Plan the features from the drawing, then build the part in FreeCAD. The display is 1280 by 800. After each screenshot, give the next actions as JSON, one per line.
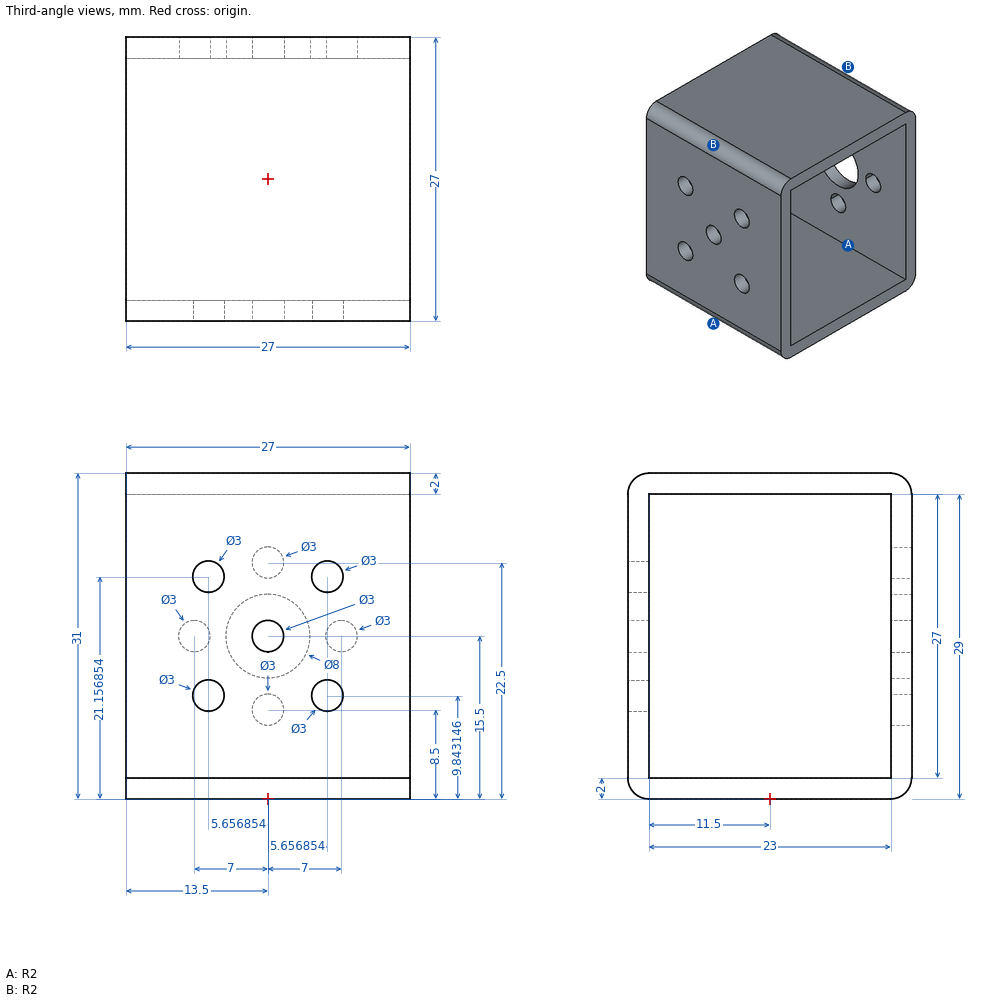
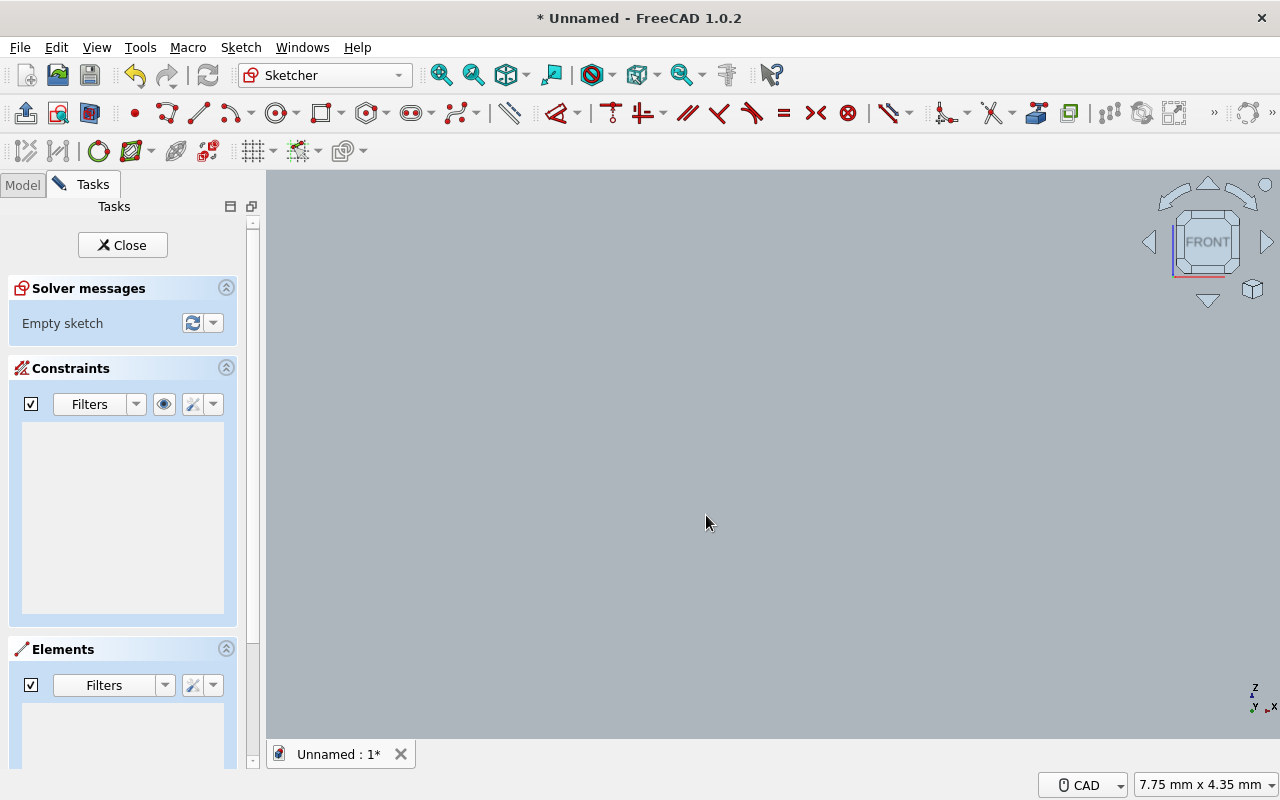
{"action": "left_click", "coordinate": [276, 114]}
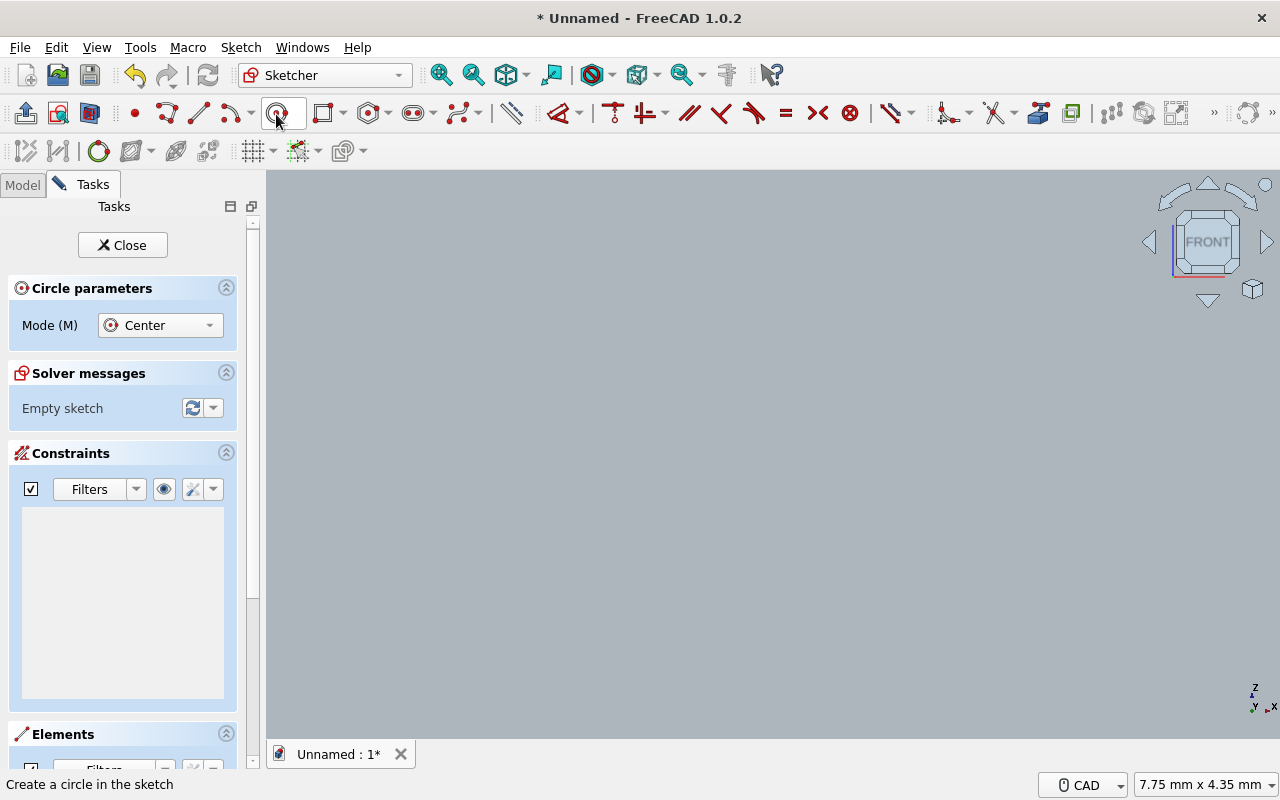
{"action": "left_click", "coordinate": [700, 451]}
{"action": "mouse_move", "coordinate": [839, 312]}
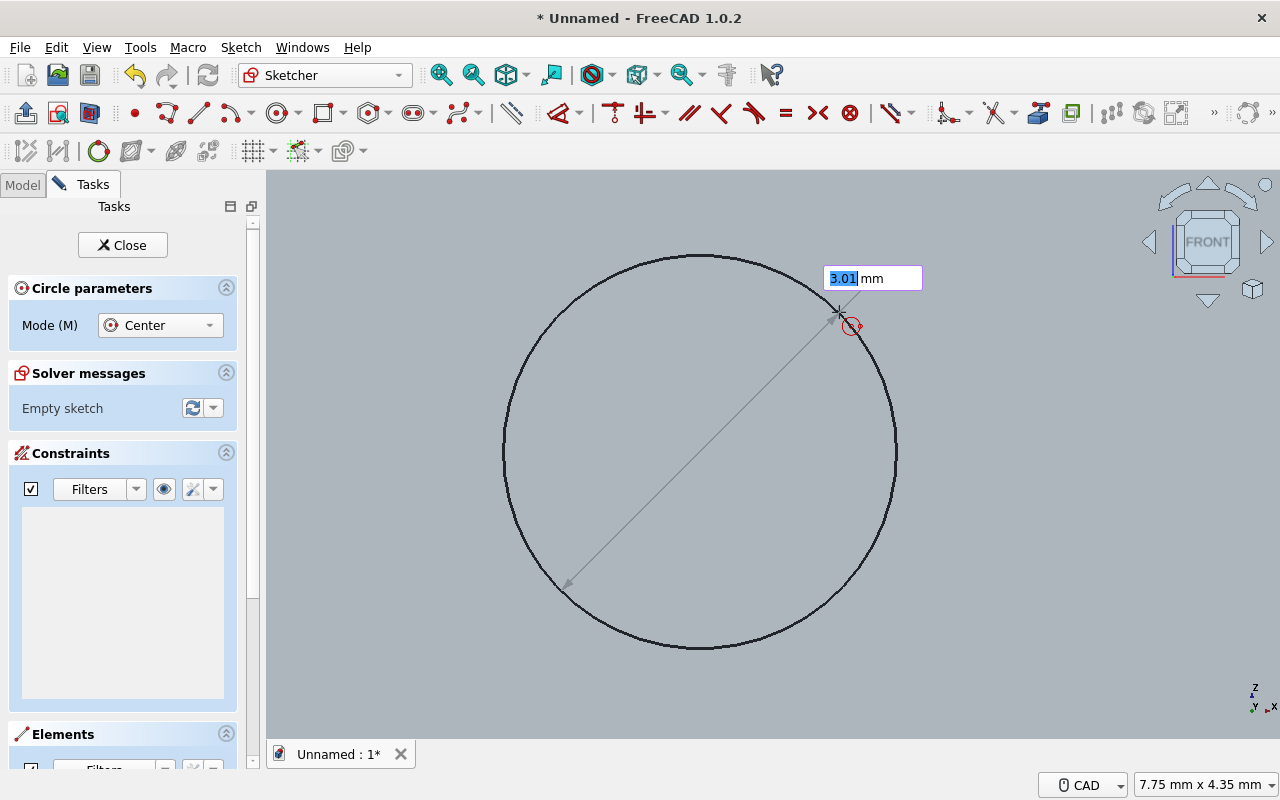
{"action": "type", "text": "3"}
{"action": "key", "text": "Return"}
{"action": "key", "text": "Escape"}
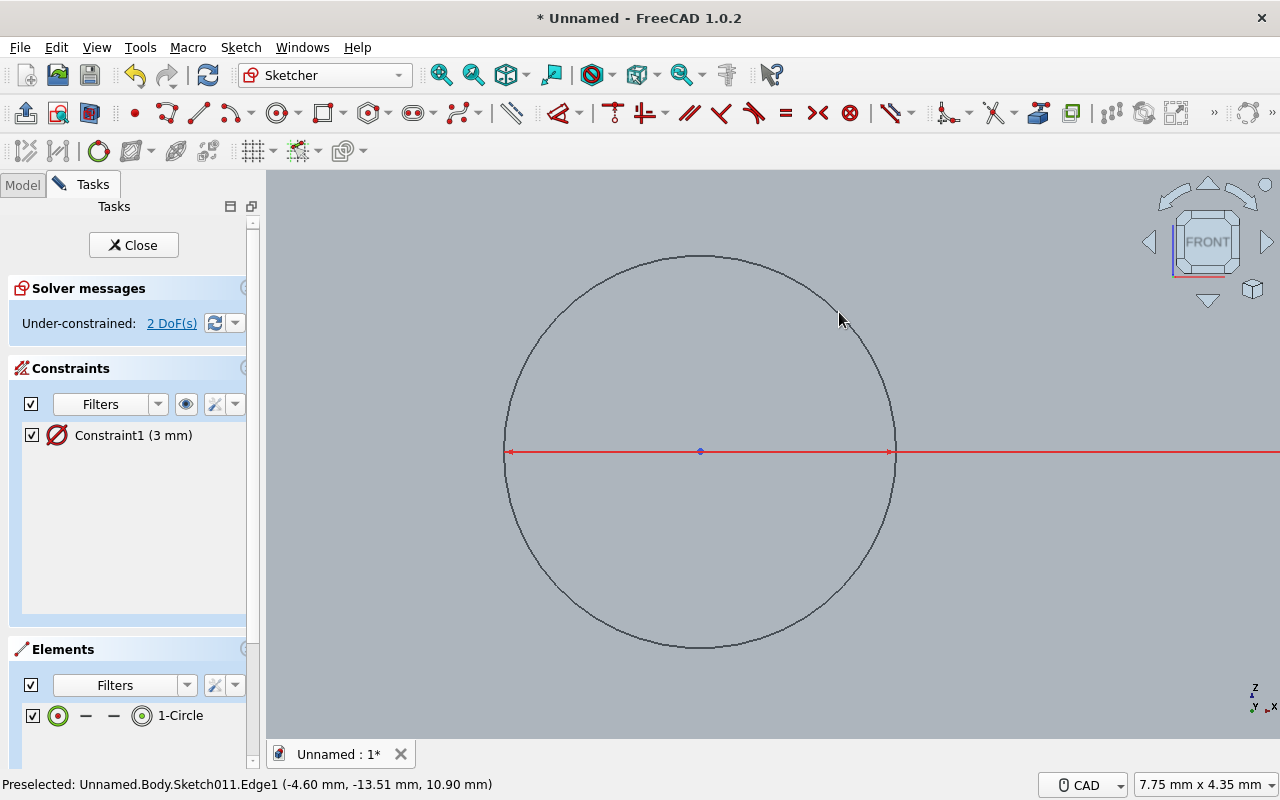
{"action": "key", "text": "d"}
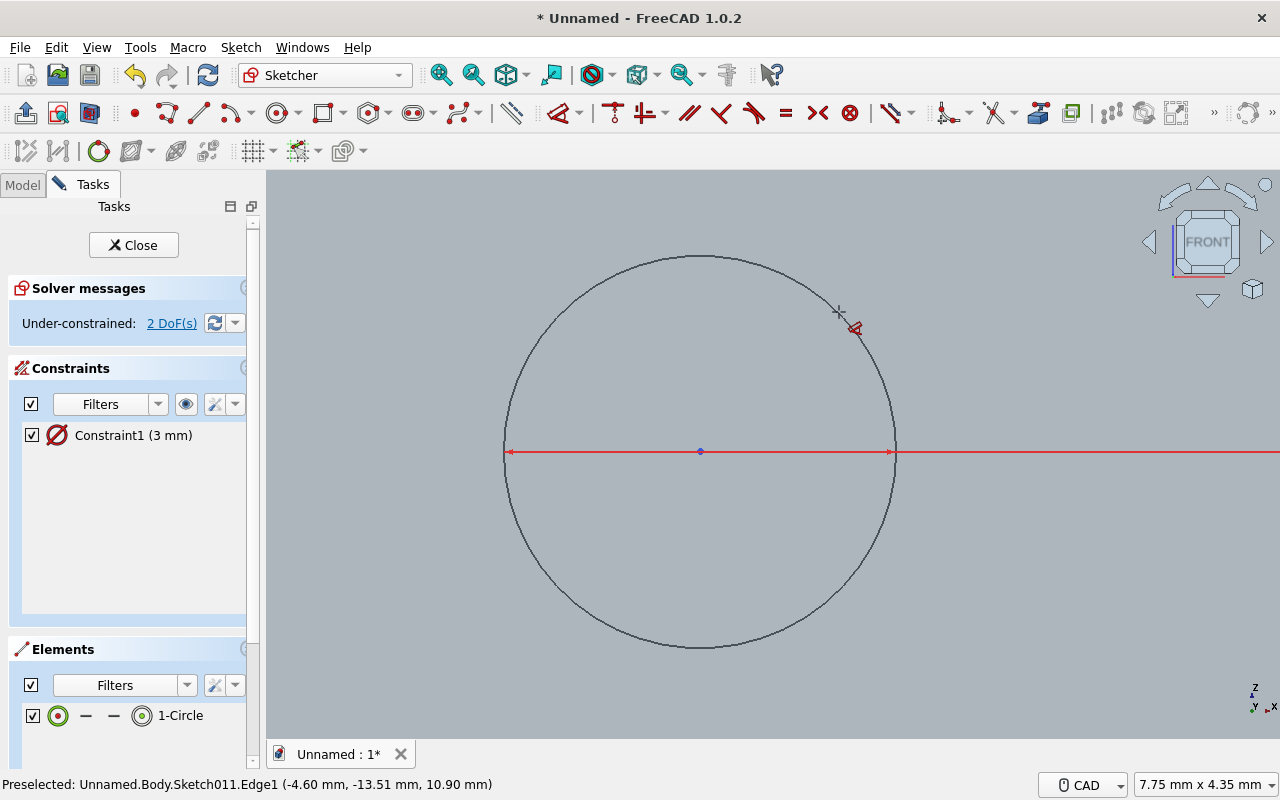
{"action": "left_click", "coordinate": [700, 452]}
{"action": "left_click", "coordinate": [907, 418]}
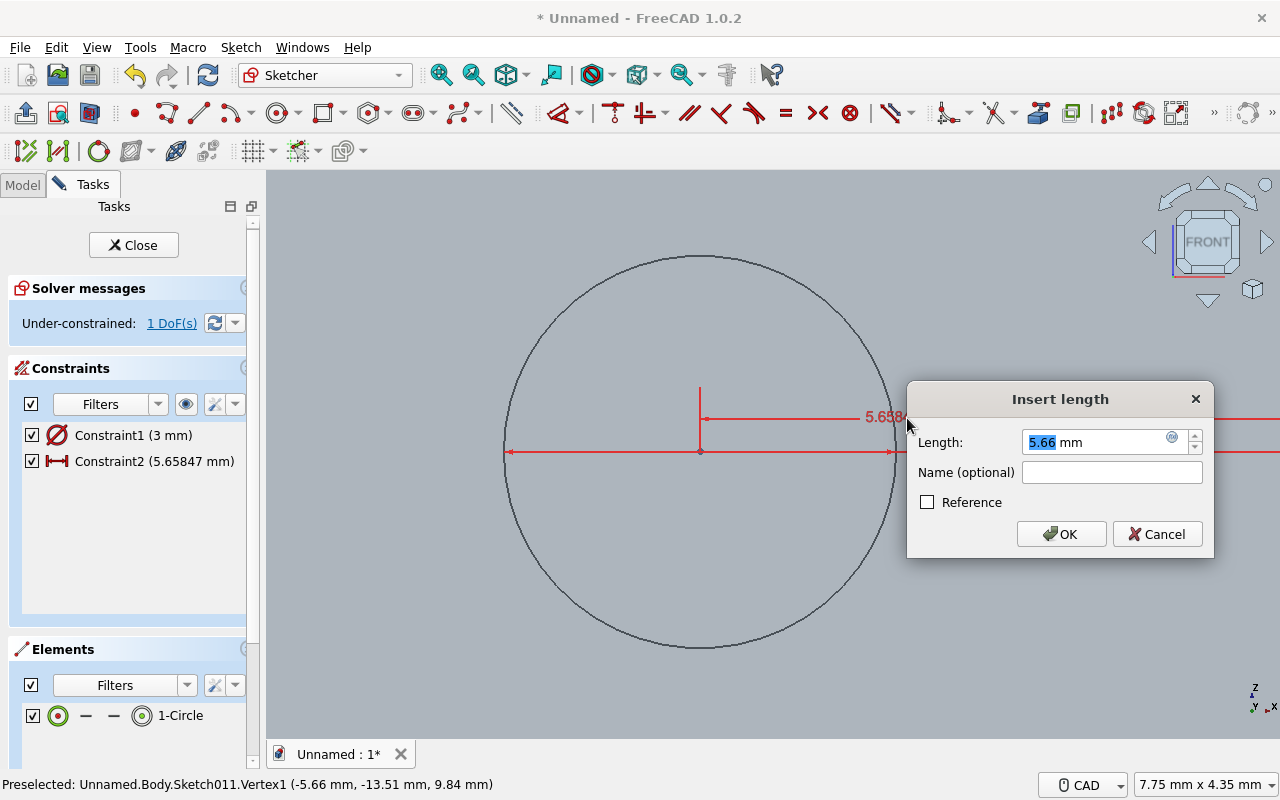
{"action": "type", "text": "5.656854"}
{"action": "key", "text": "Return"}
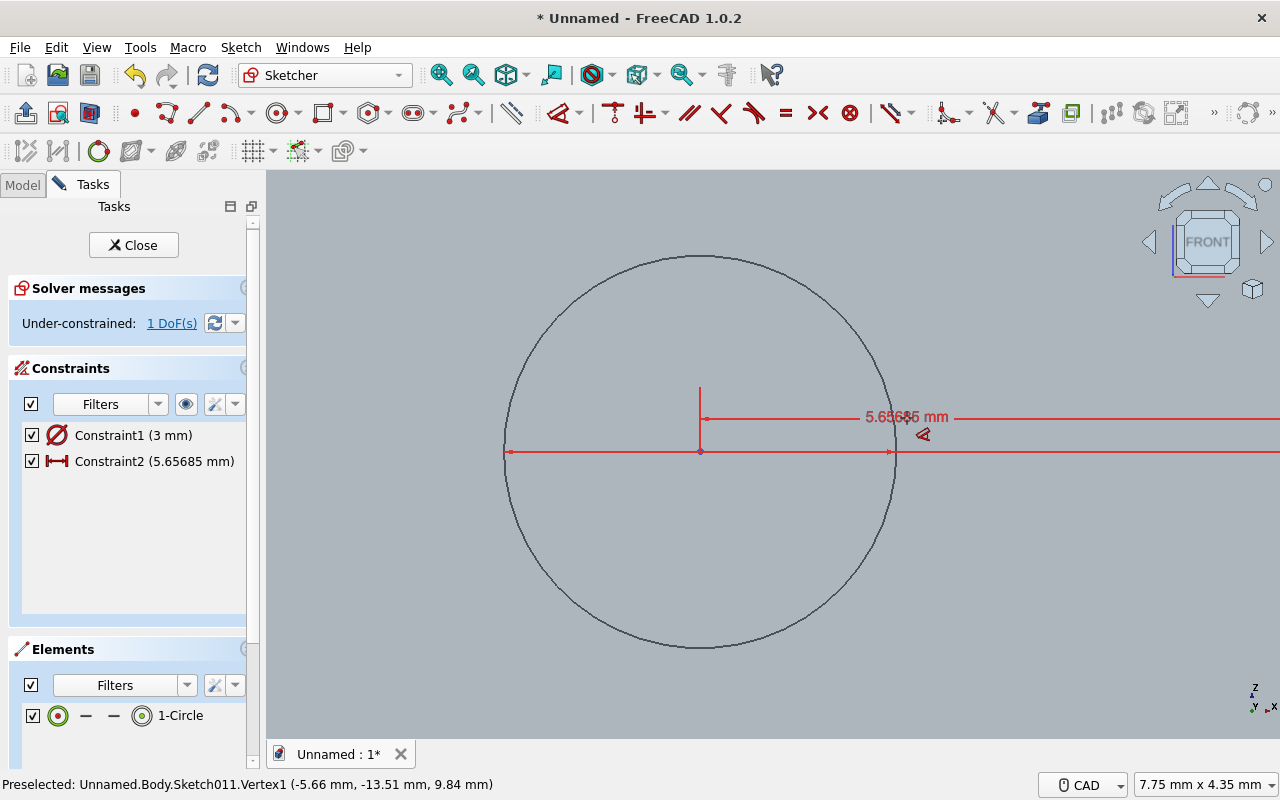
{"action": "left_click", "coordinate": [700, 452]}
{"action": "left_click", "coordinate": [666, 581]}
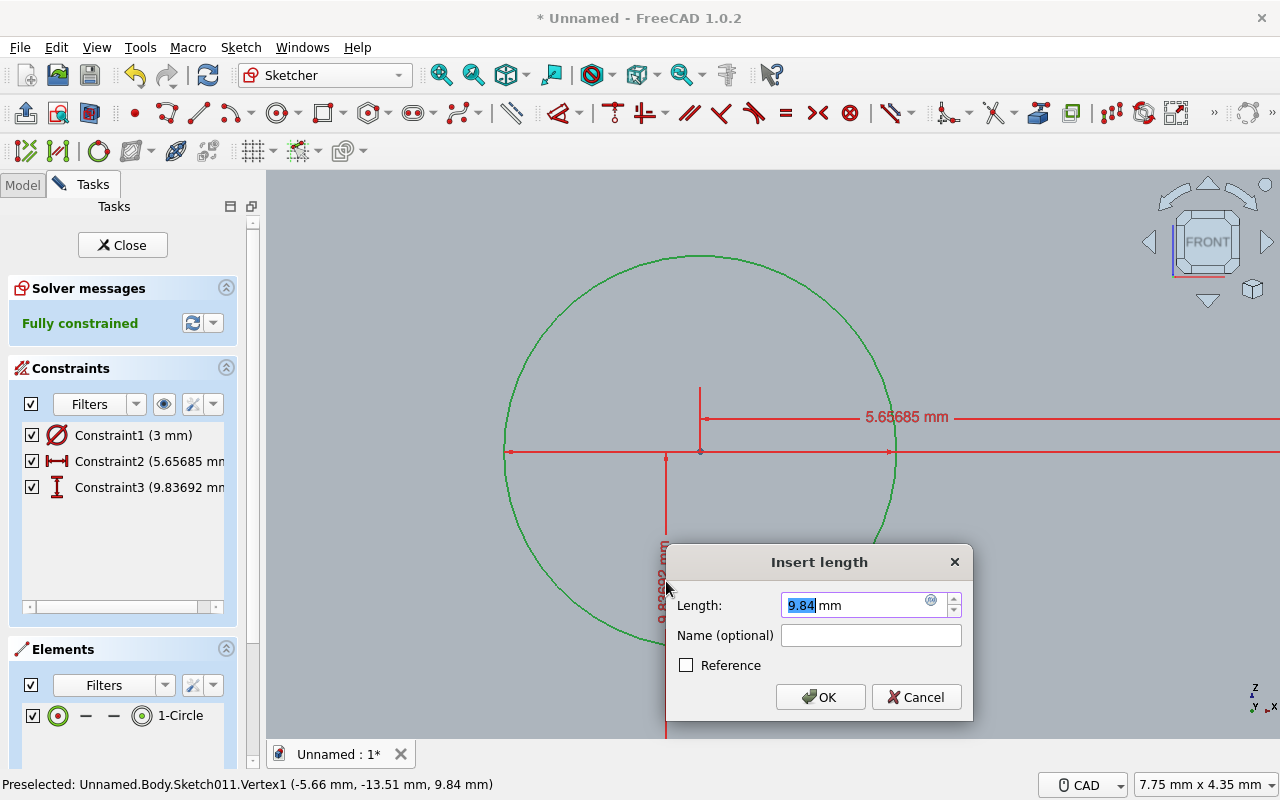
{"action": "type", "text": "9.843146"}
{"action": "key", "text": "Return"}
{"action": "key", "text": "Escape"}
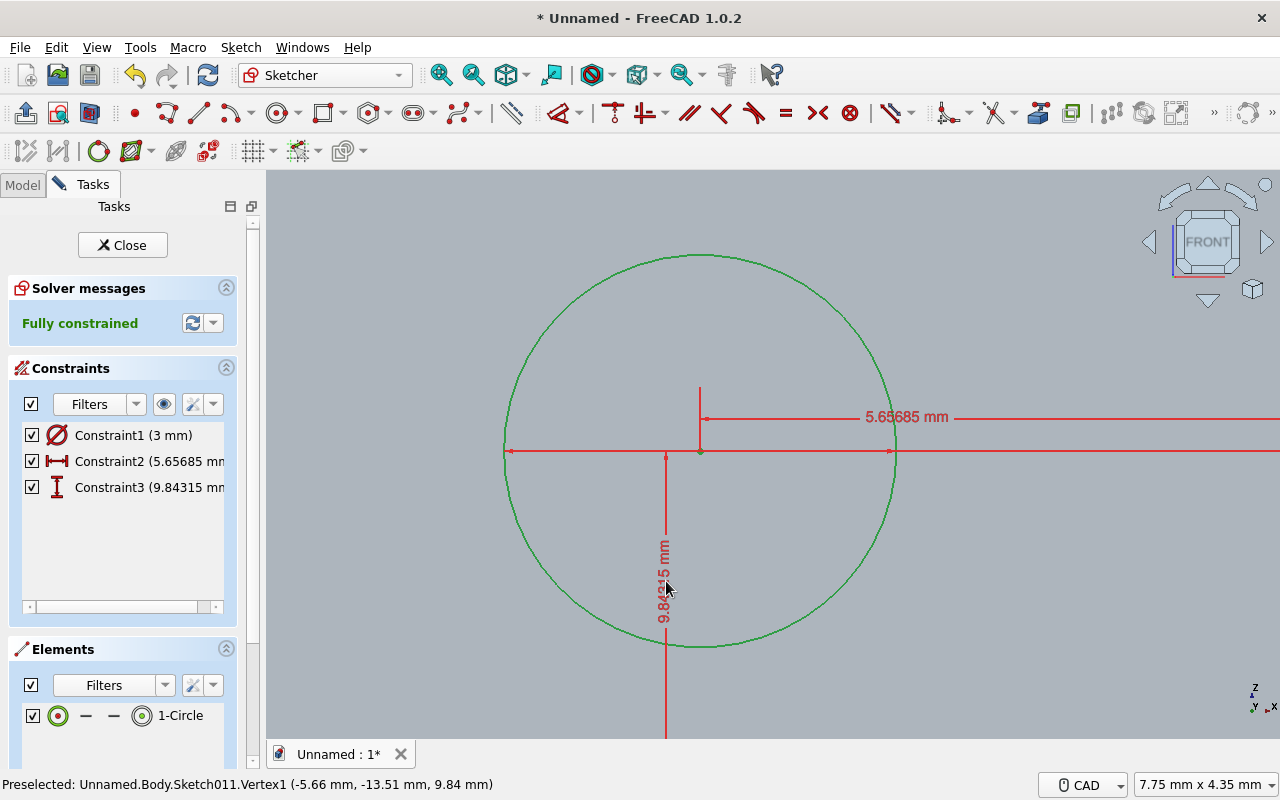
{"action": "left_click", "coordinate": [123, 245]}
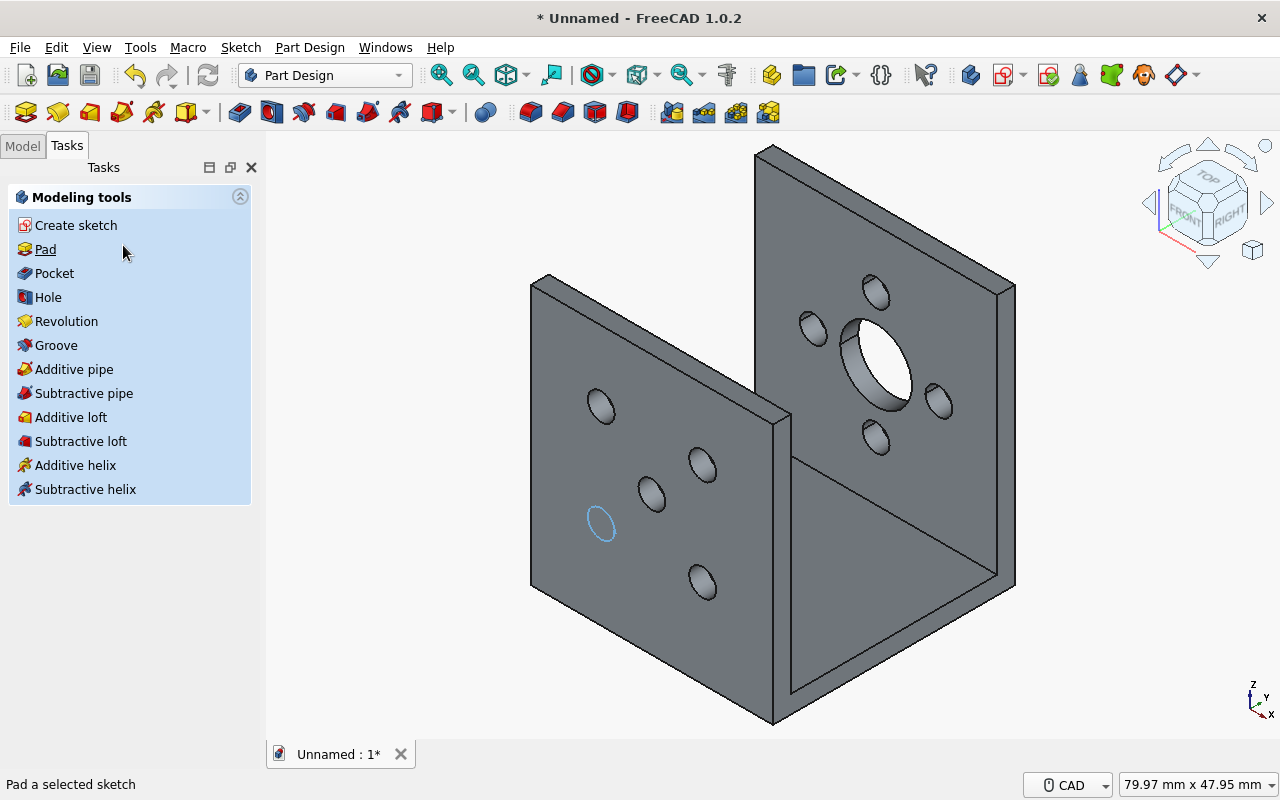
{"action": "left_click", "coordinate": [240, 112]}